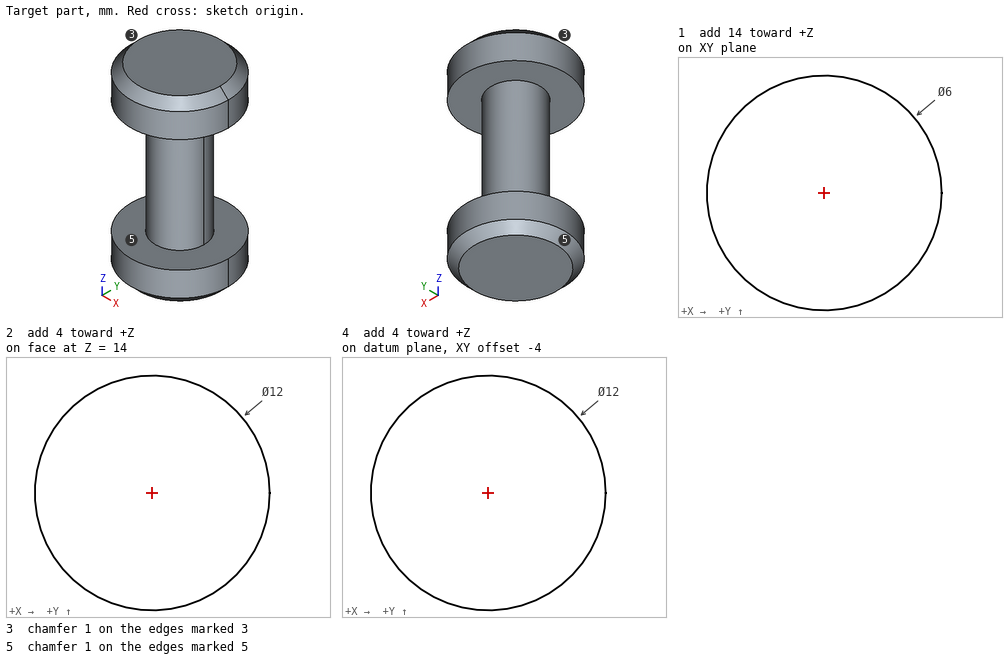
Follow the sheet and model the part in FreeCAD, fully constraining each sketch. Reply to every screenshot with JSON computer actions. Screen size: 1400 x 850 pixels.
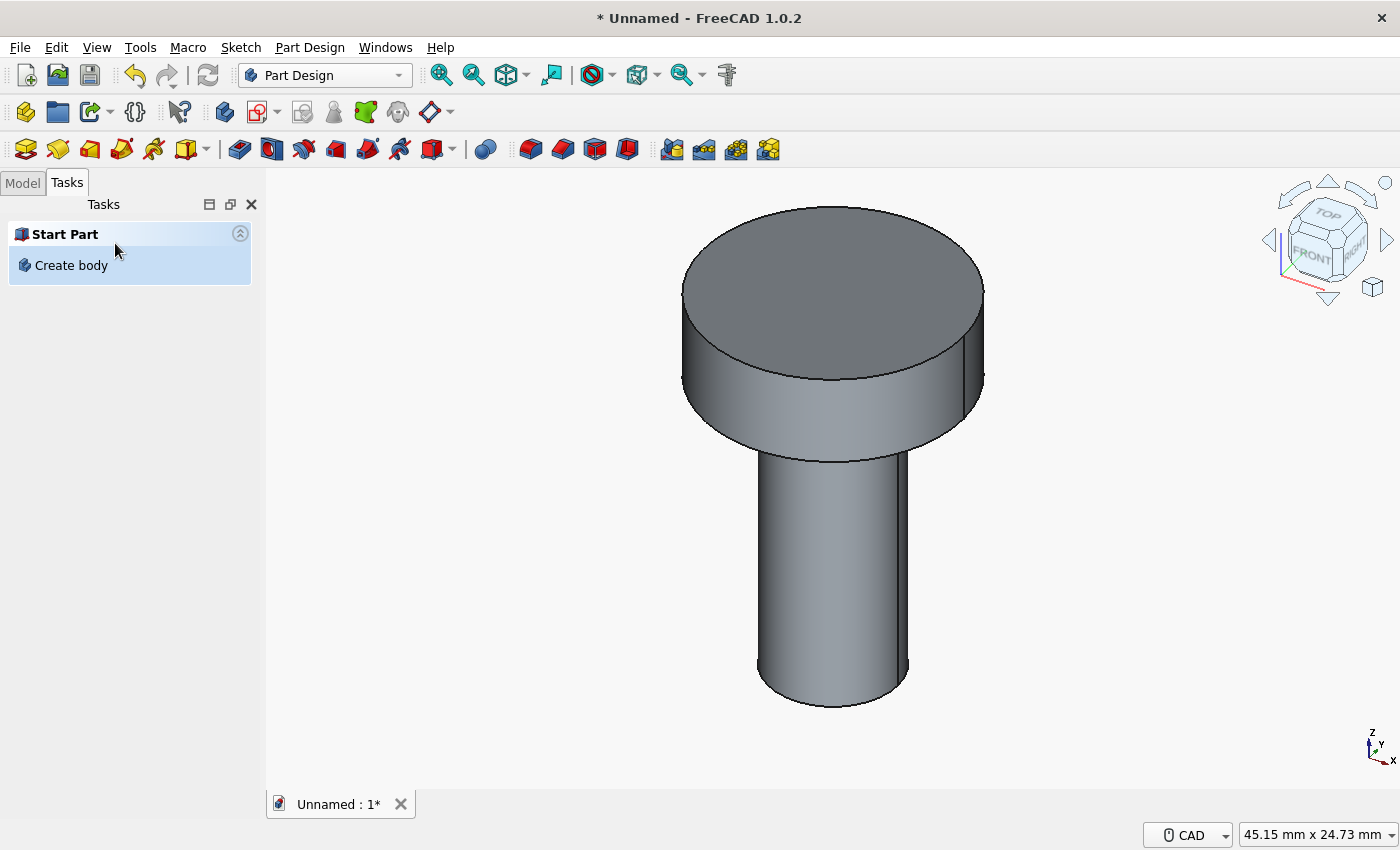
{"action": "left_click", "coordinate": [683, 301]}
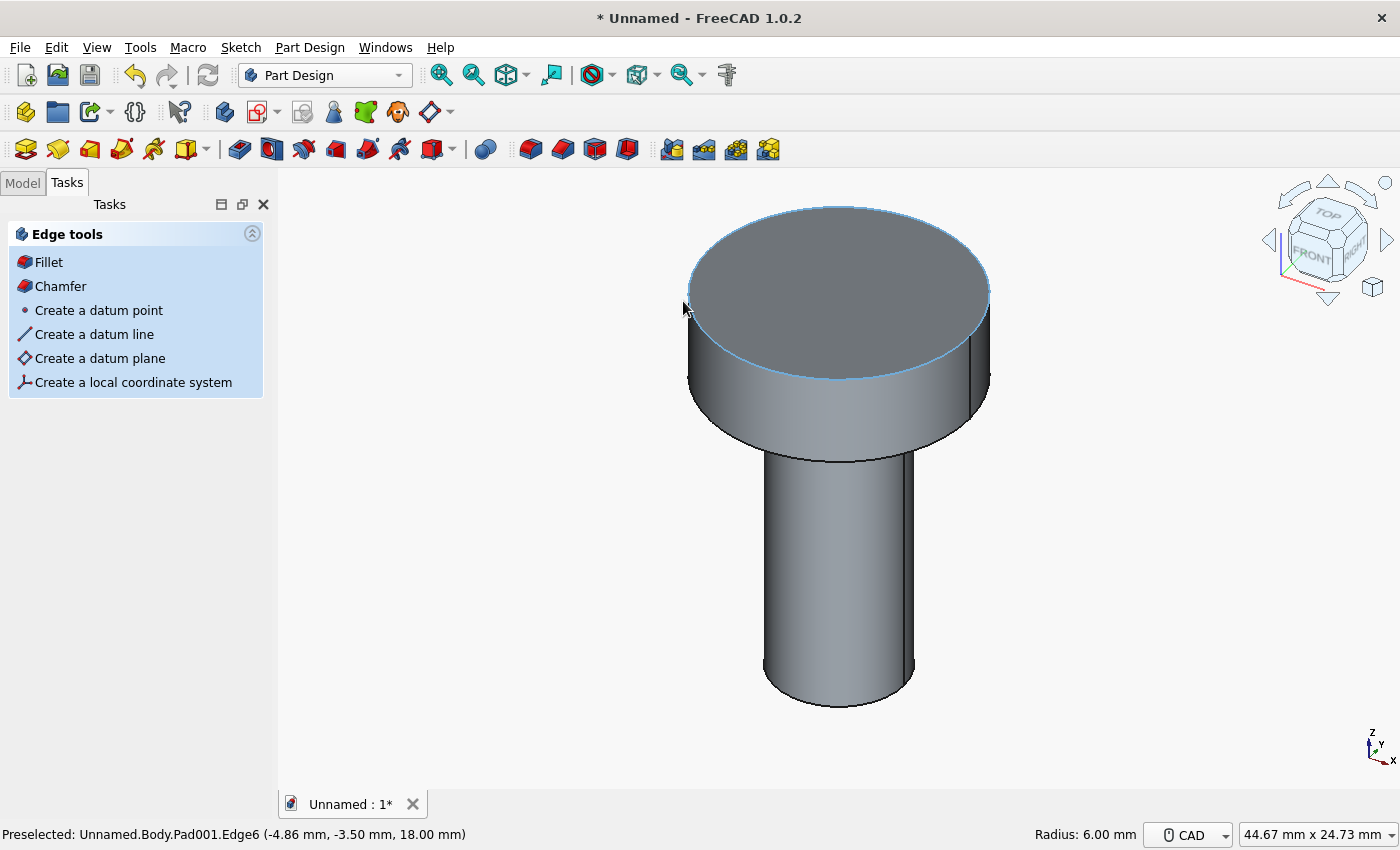
{"action": "left_click", "coordinate": [564, 150]}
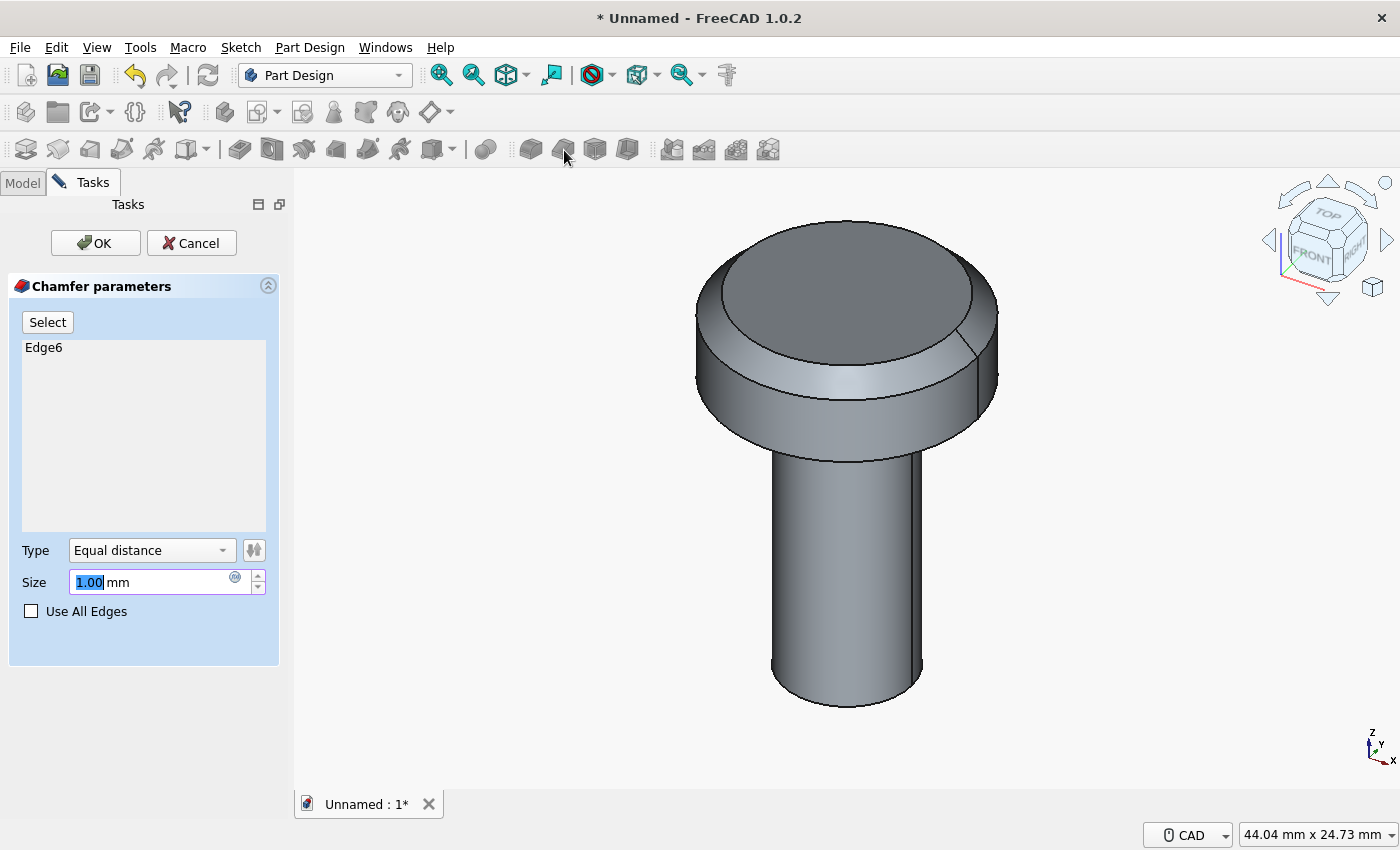
{"action": "type", "text": "1"}
{"action": "key", "text": "Tab"}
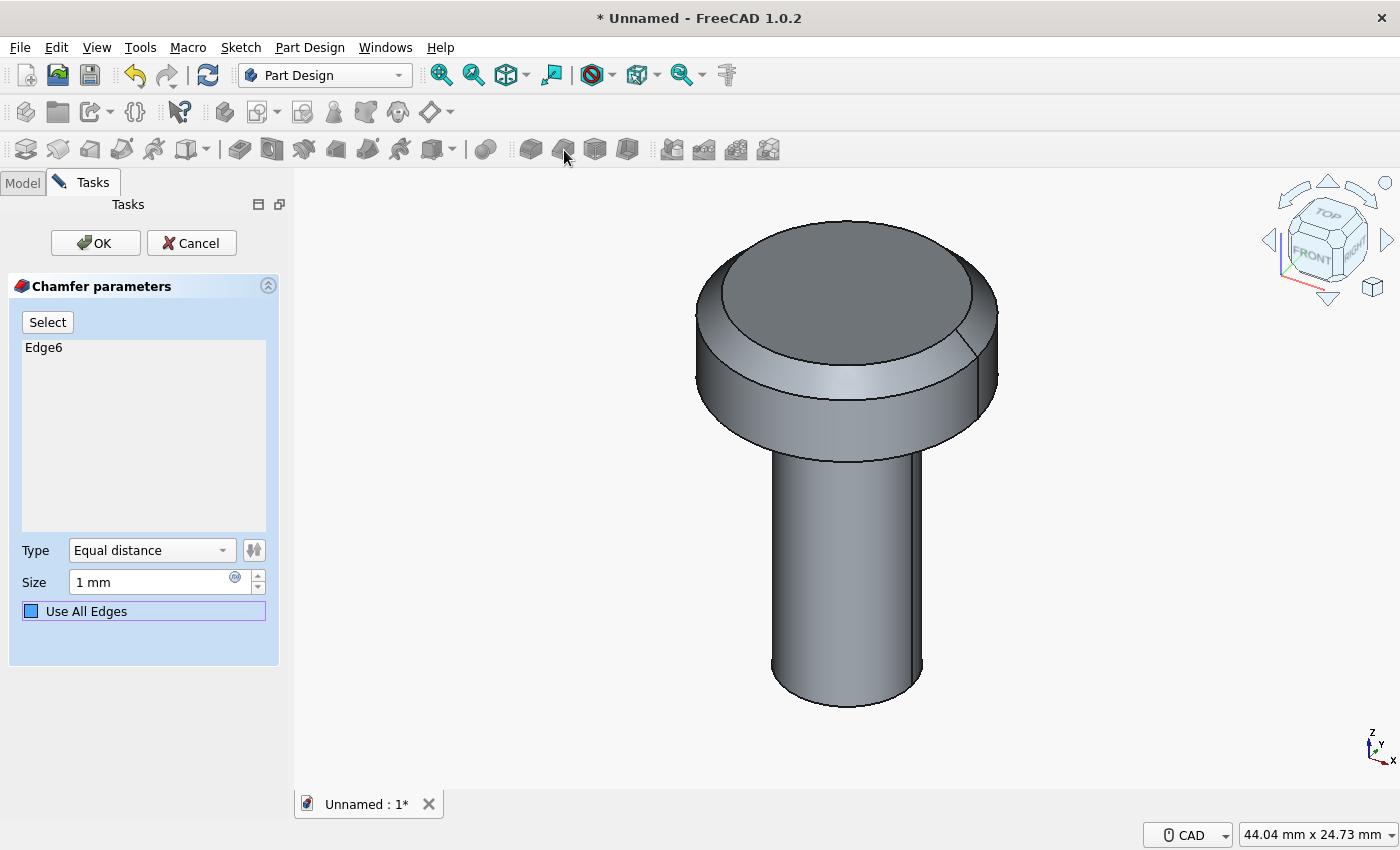
{"action": "left_click", "coordinate": [96, 243]}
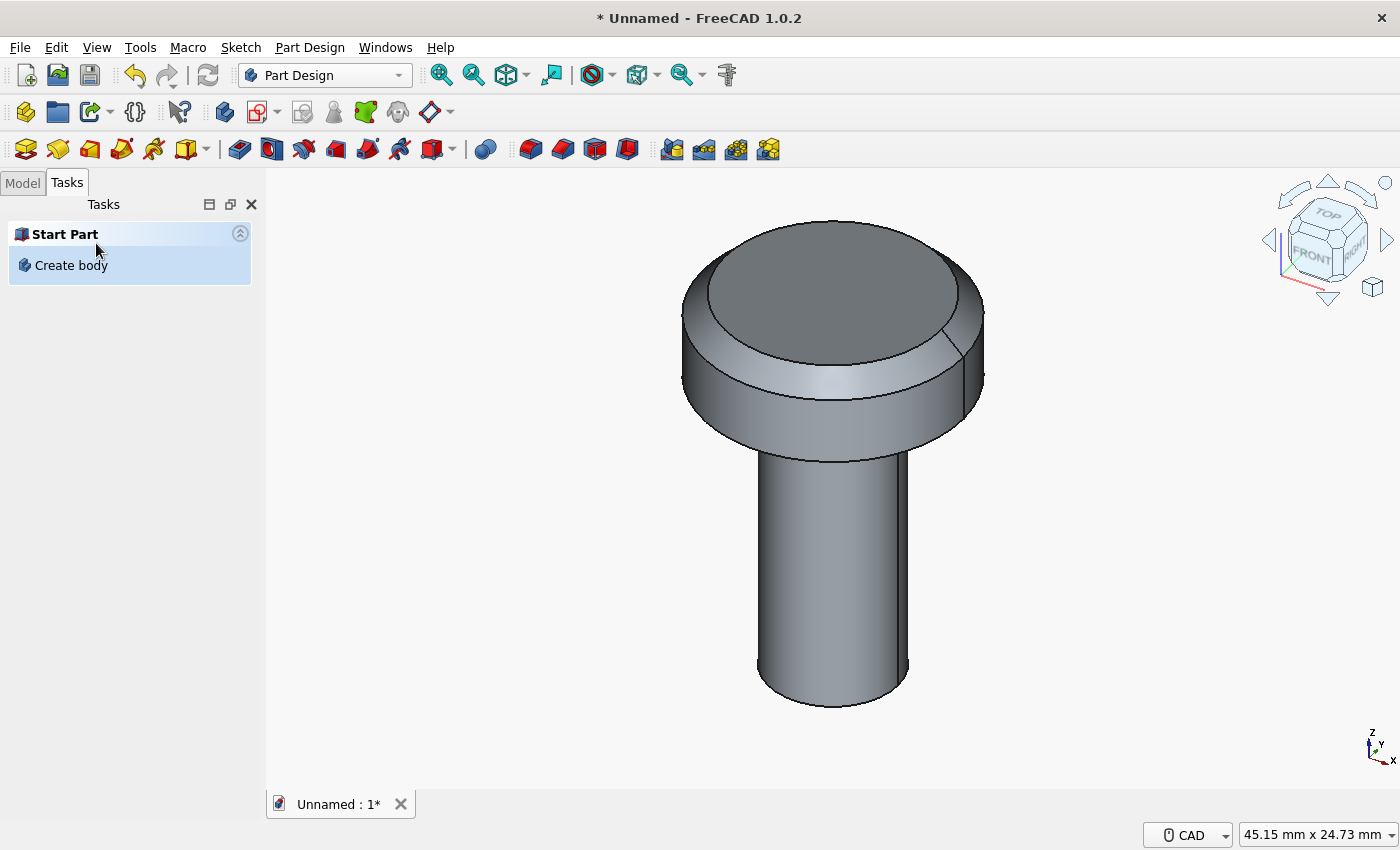
{"action": "left_click", "coordinate": [23, 182]}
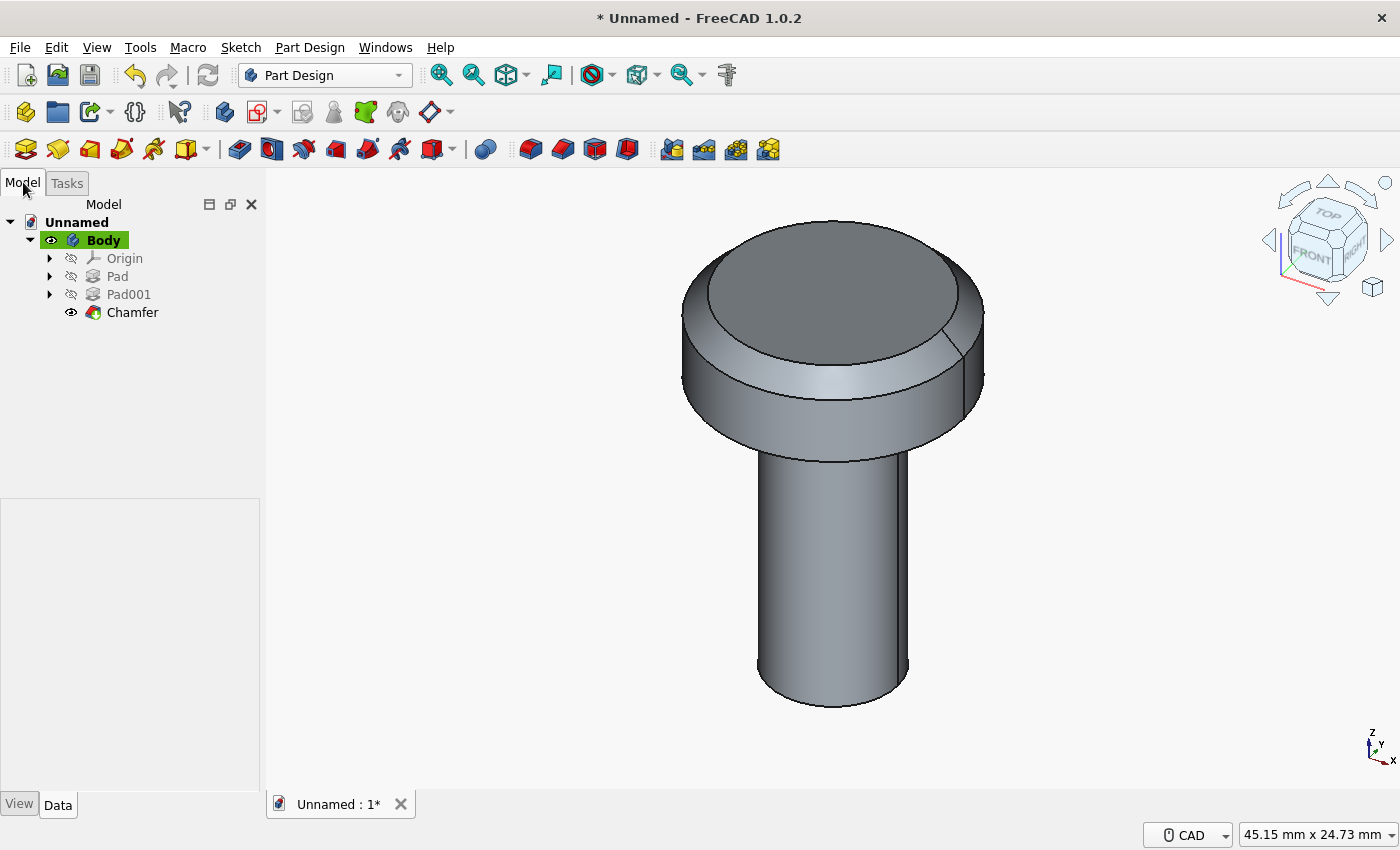
{"action": "left_click", "coordinate": [50, 258]}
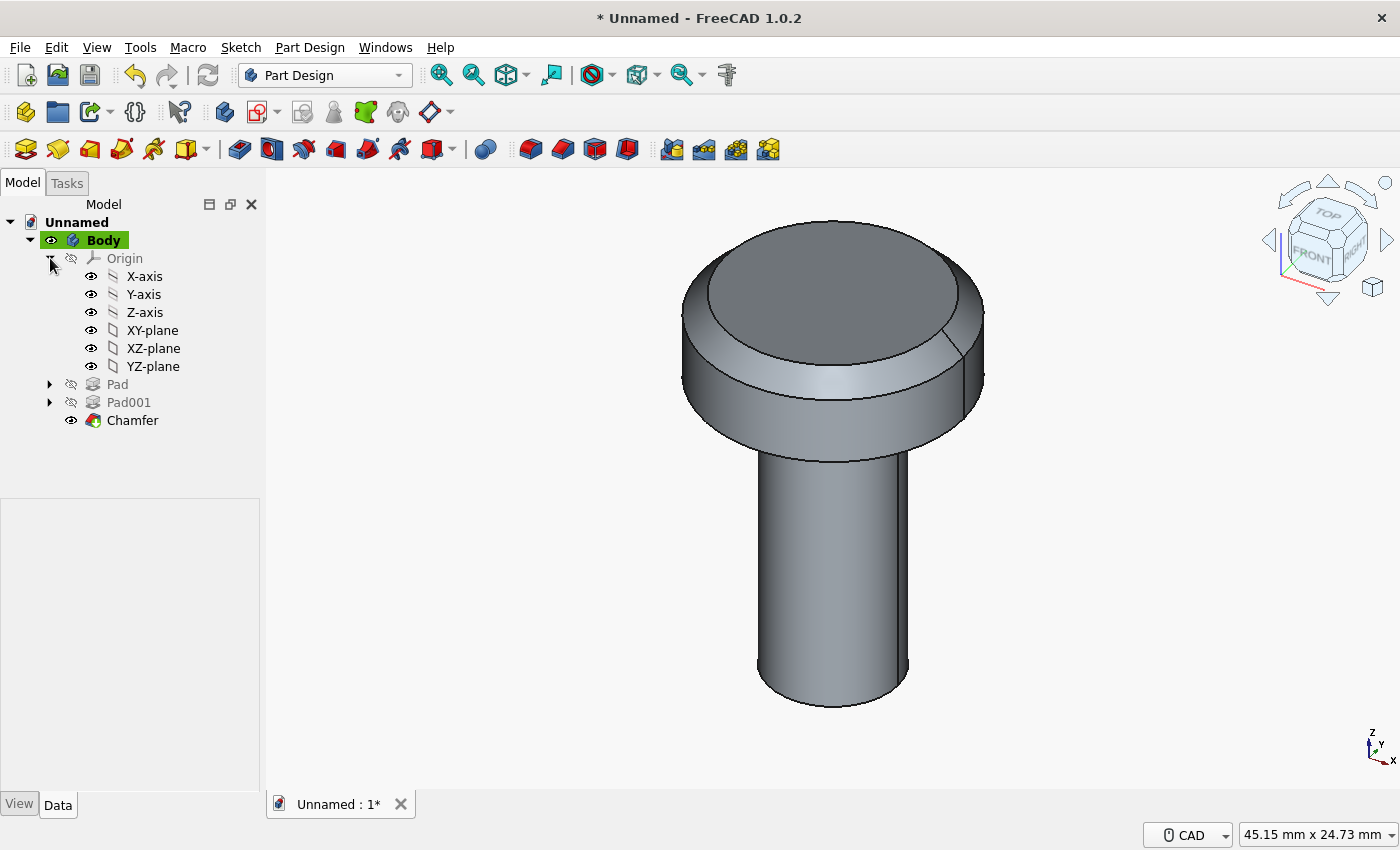
{"action": "left_click", "coordinate": [136, 330]}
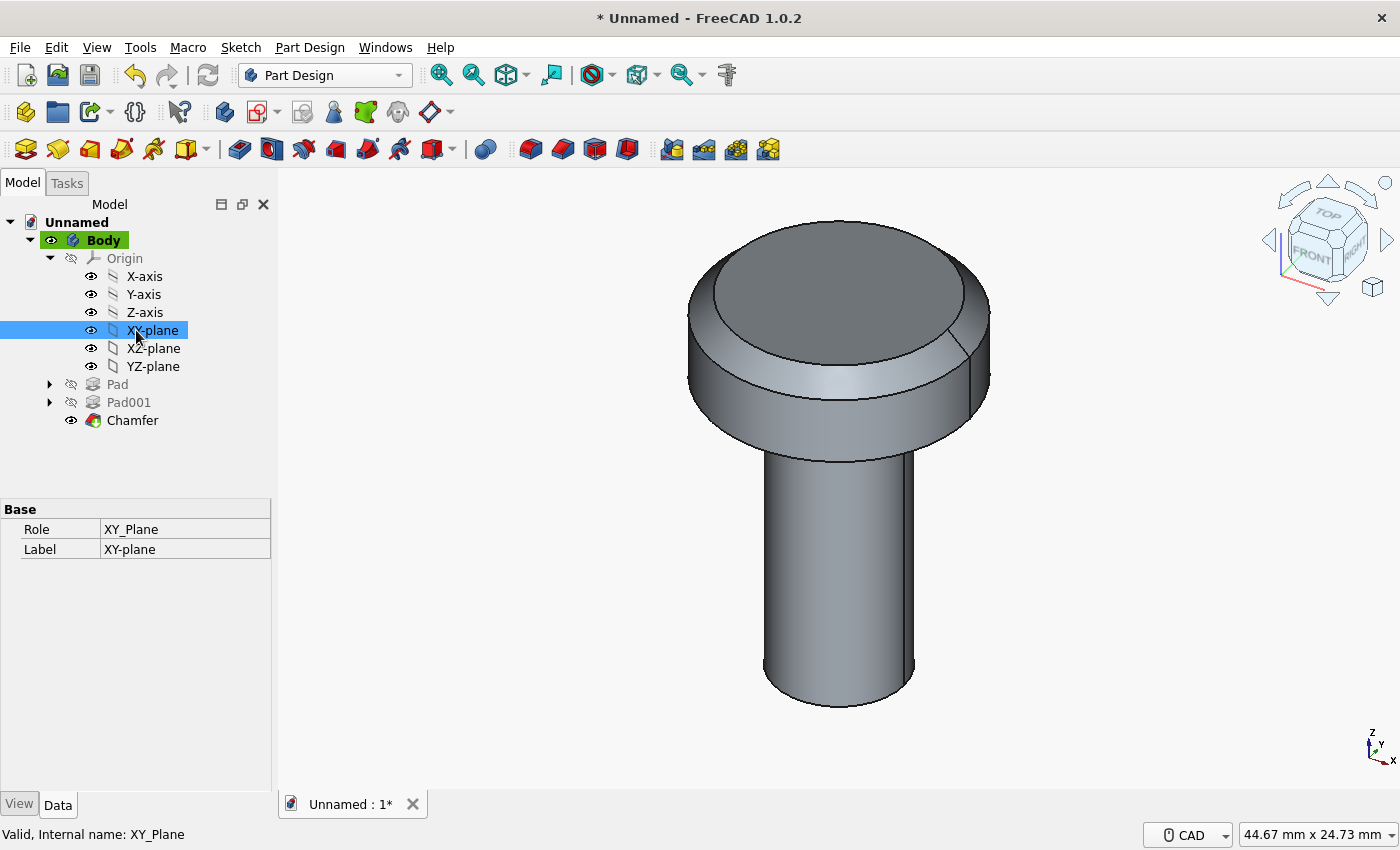
{"action": "left_click", "coordinate": [430, 112]}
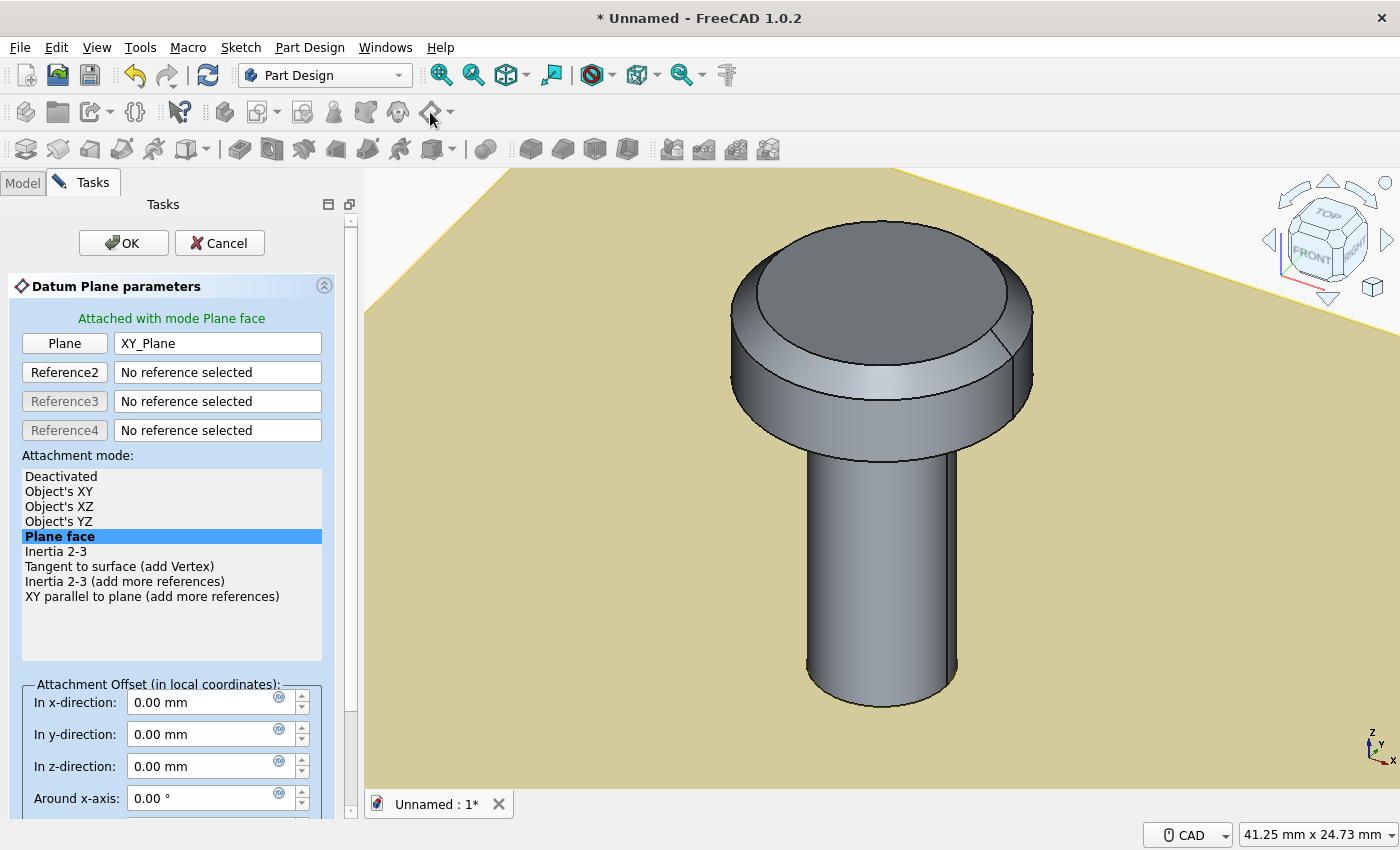
{"action": "triple_click", "coordinate": [210, 766]}